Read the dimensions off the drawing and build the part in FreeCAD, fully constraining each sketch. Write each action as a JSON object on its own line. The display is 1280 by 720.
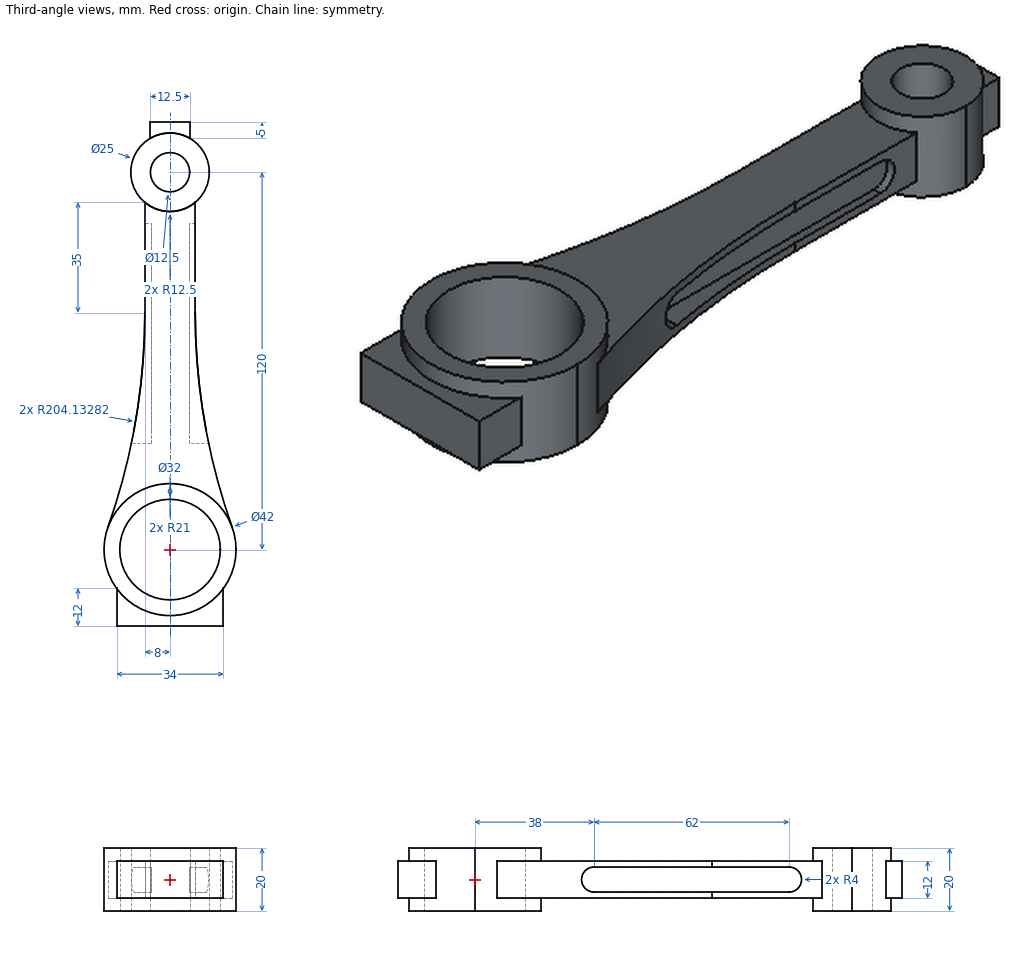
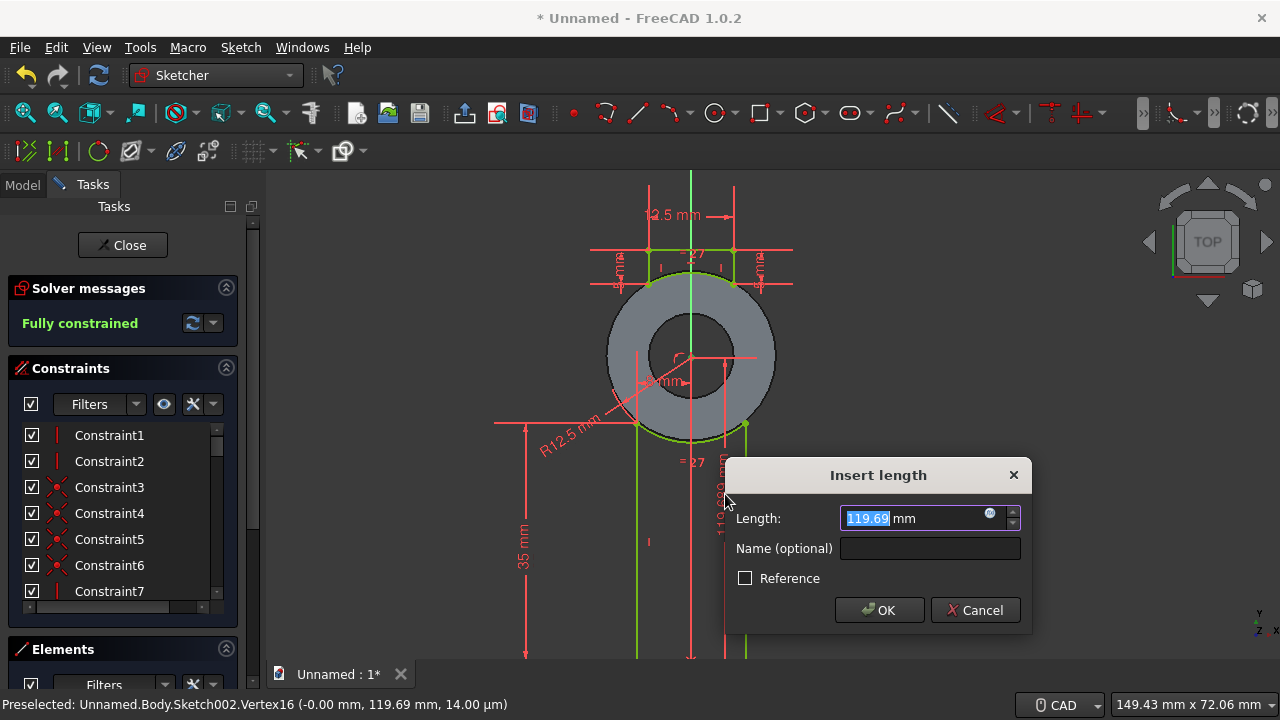
{"action": "type", "text": "120"}
{"action": "key", "text": "Return"}
{"action": "key", "text": "Escape"}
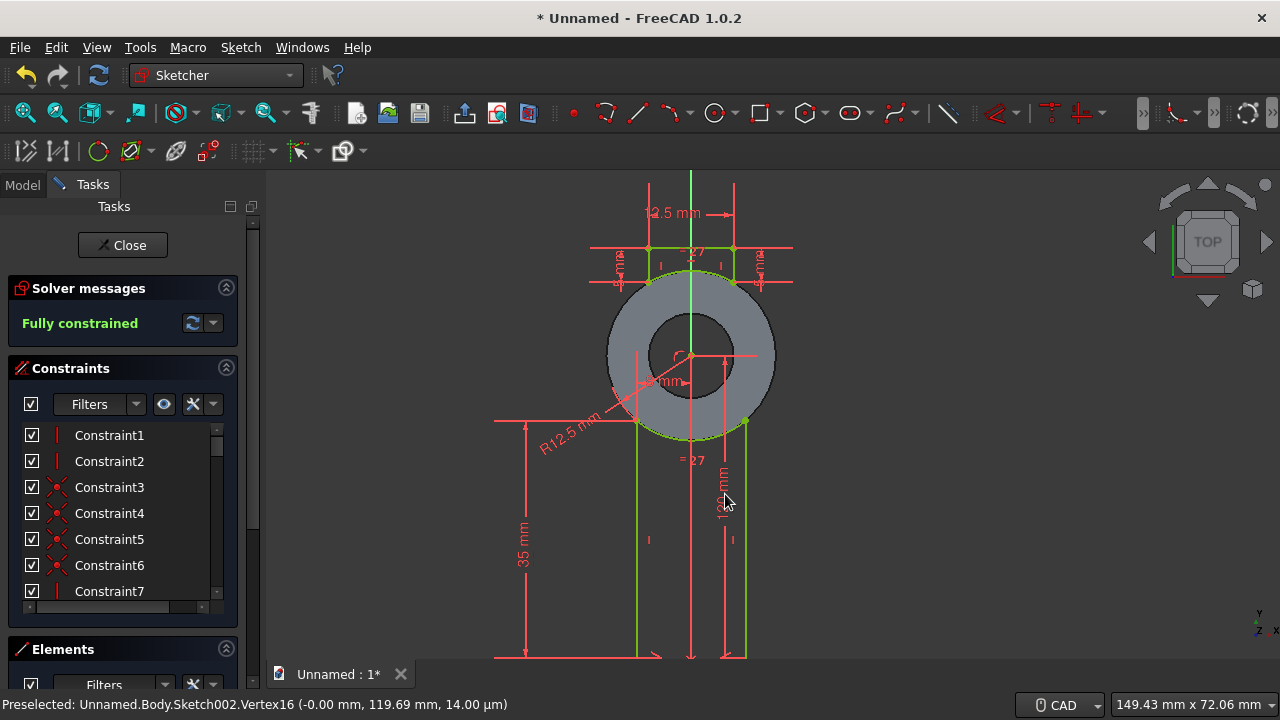
{"action": "left_click", "coordinate": [123, 245]}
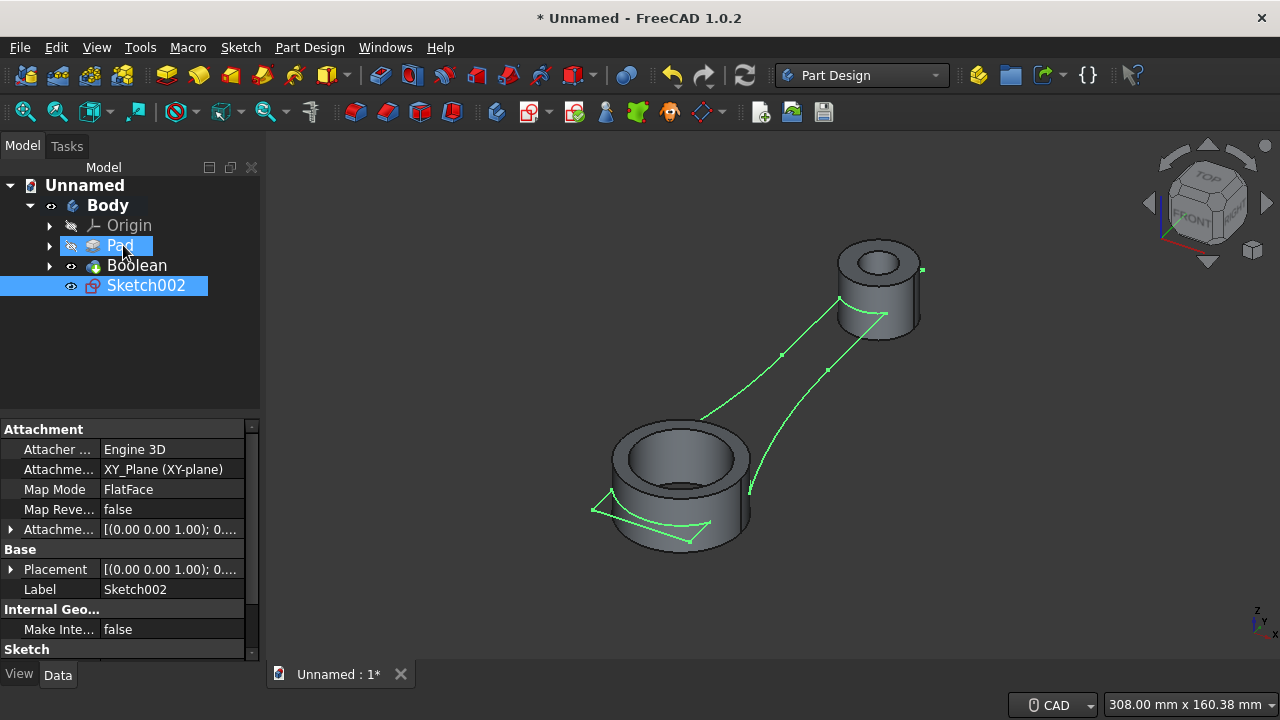
{"action": "left_click", "coordinate": [168, 76]}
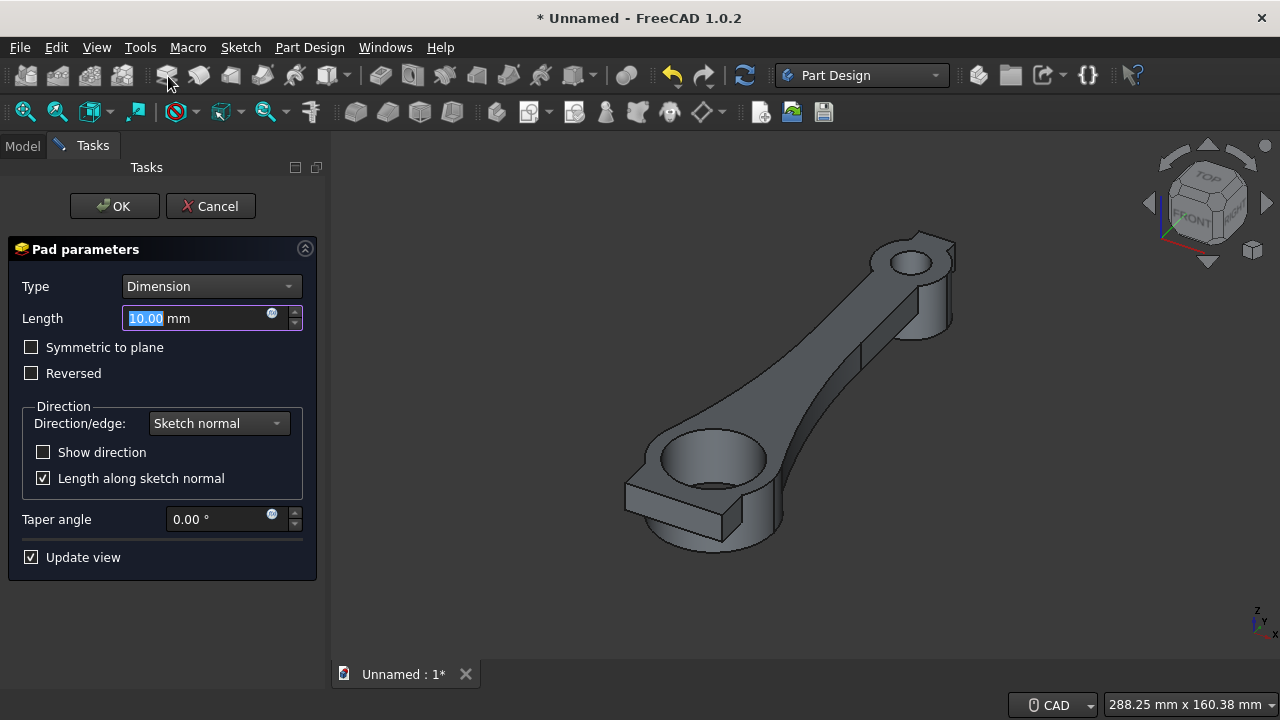
{"action": "type", "text": "12"}
{"action": "key", "text": "Tab"}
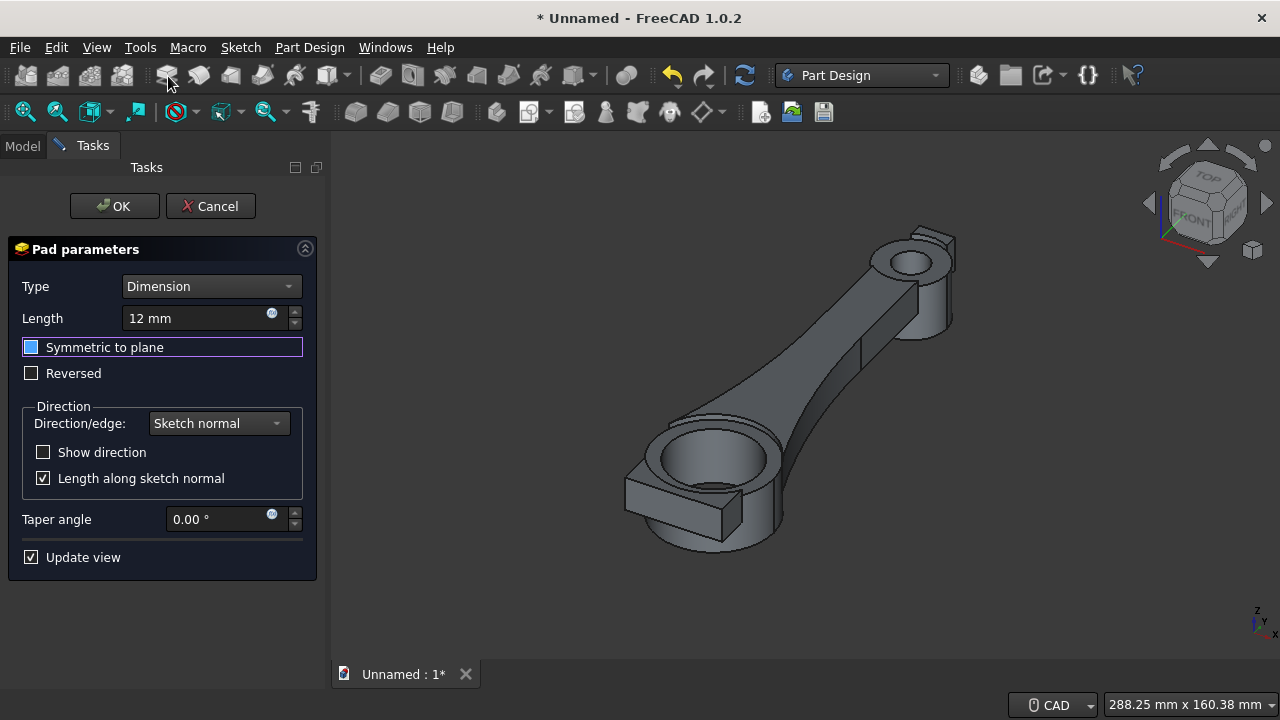
{"action": "left_click", "coordinate": [30, 347]}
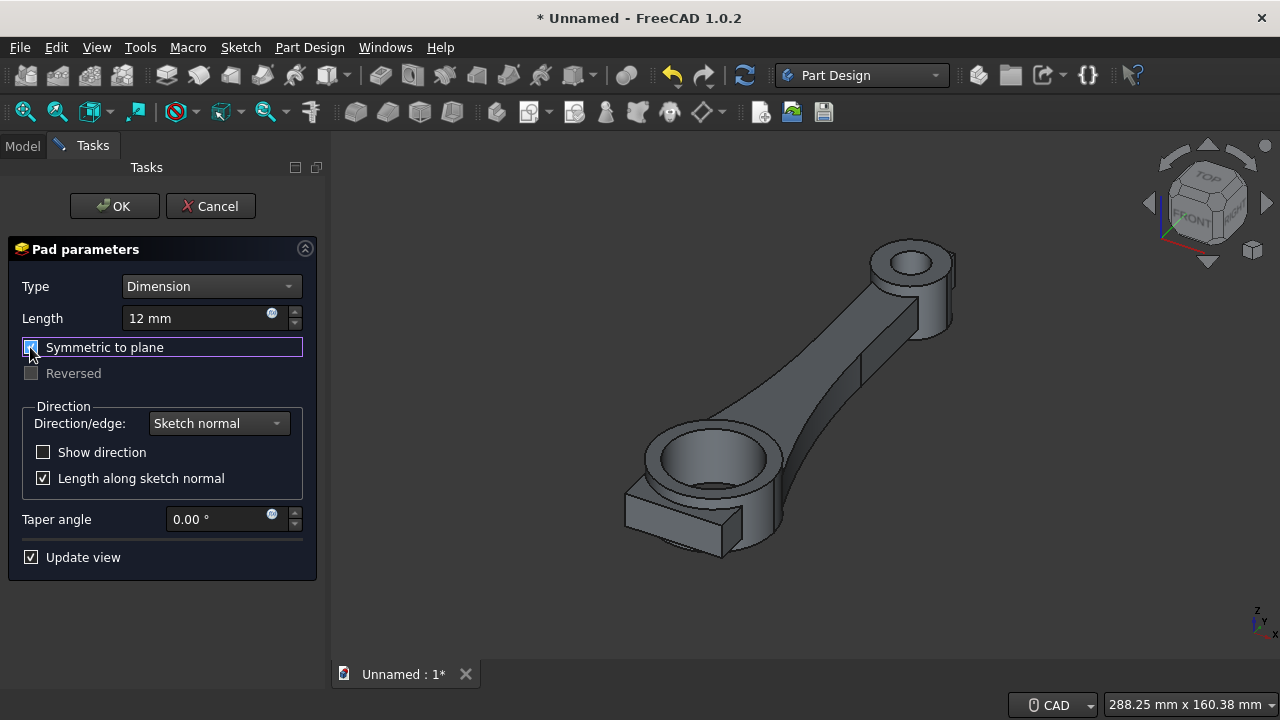
{"action": "left_click", "coordinate": [115, 206]}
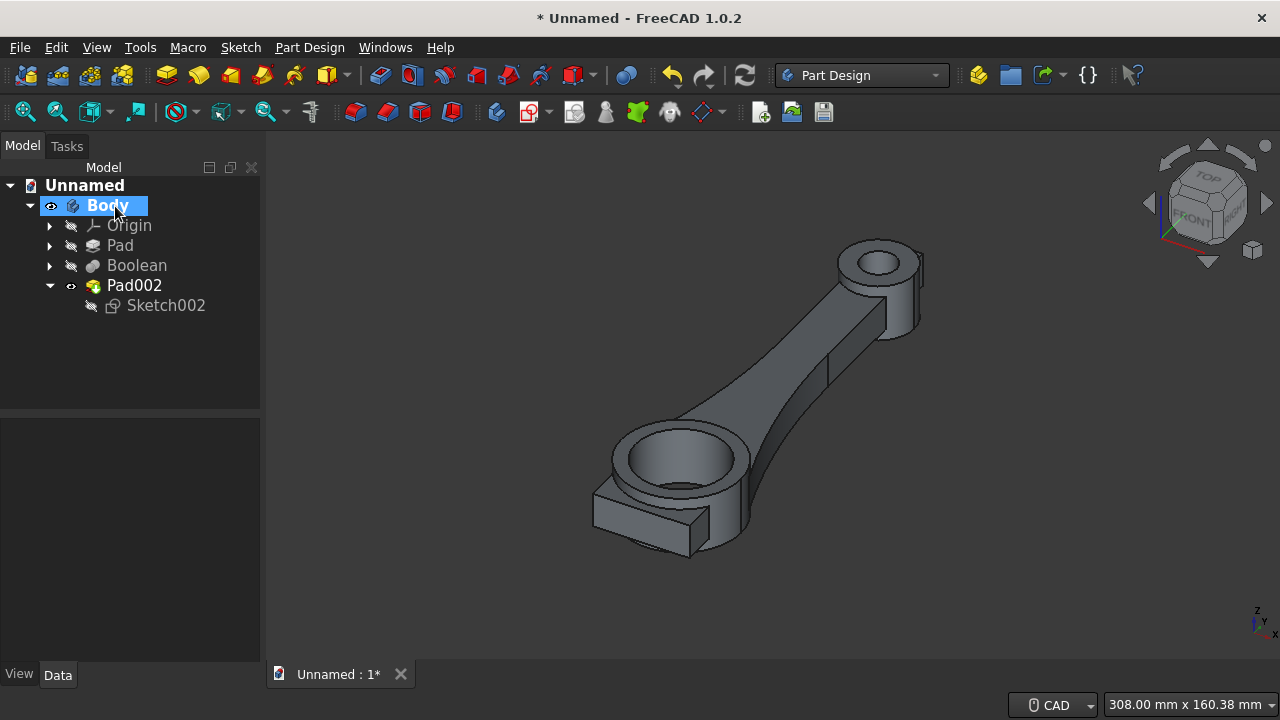
{"action": "left_click", "coordinate": [50, 226]}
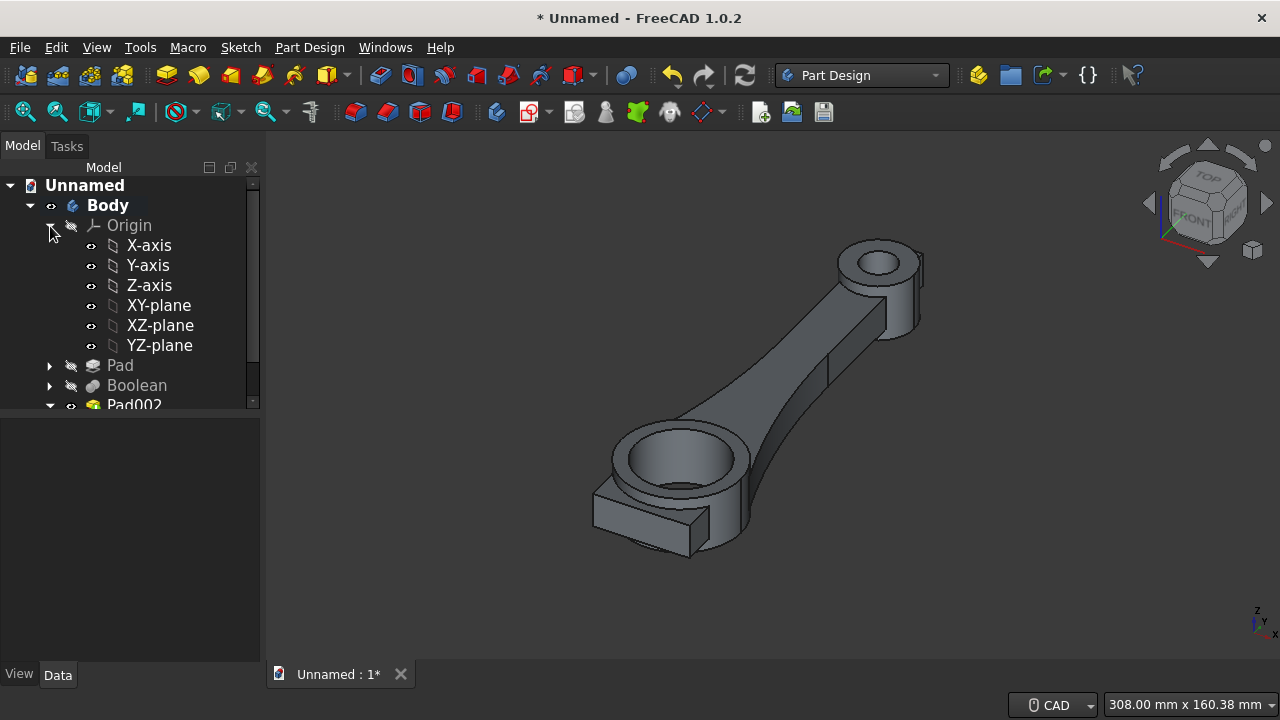
{"action": "left_click", "coordinate": [136, 346]}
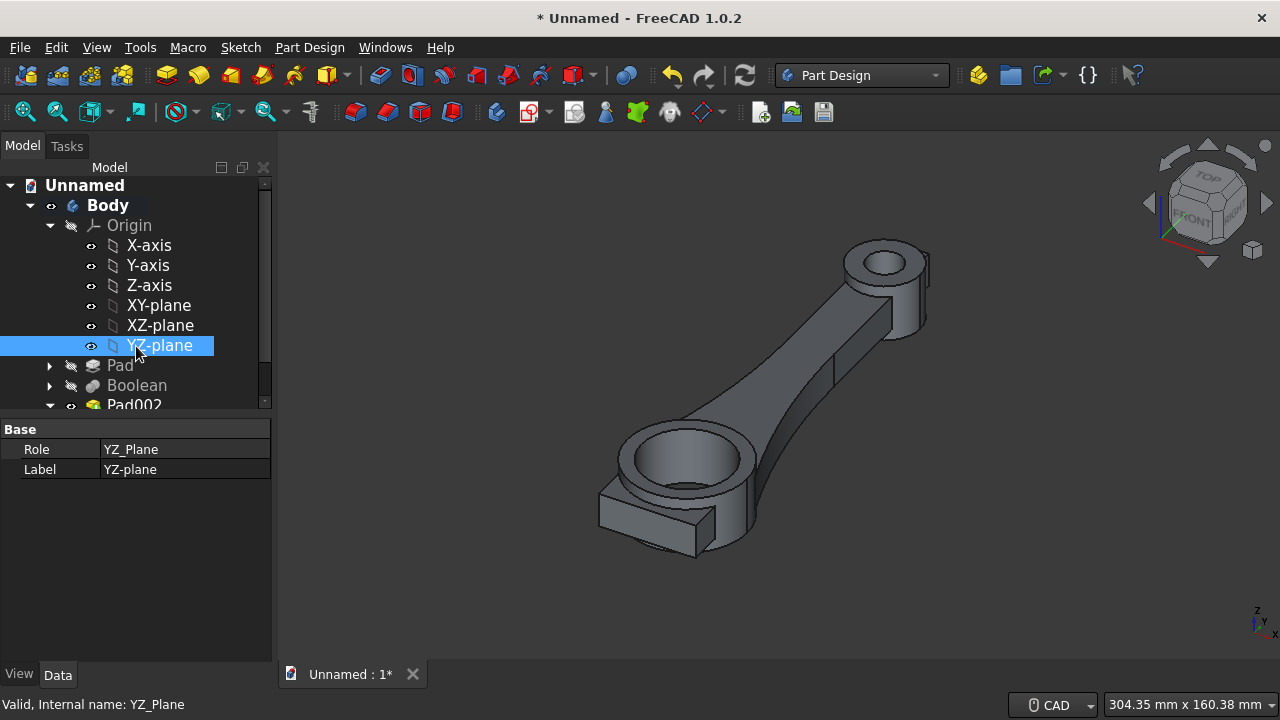
{"action": "left_click", "coordinate": [702, 112]}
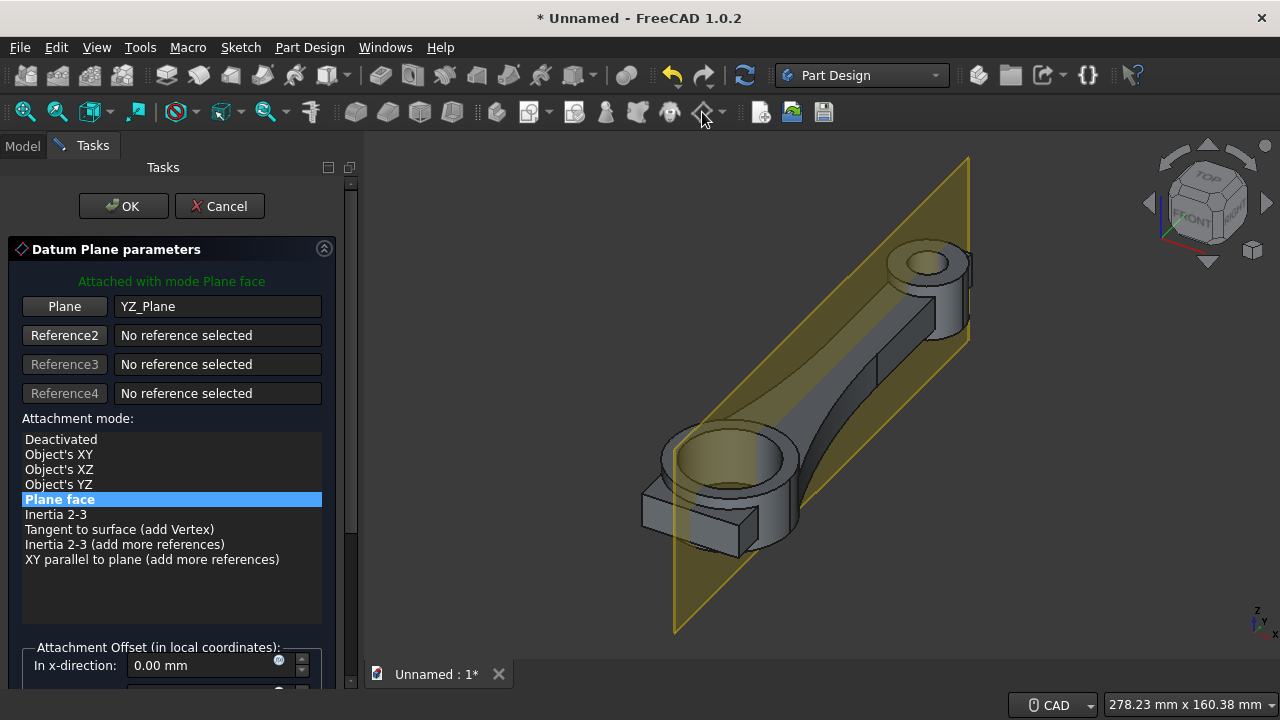
{"action": "scroll", "coordinate": [351, 432], "scroll_direction": "down", "scroll_amount": 2}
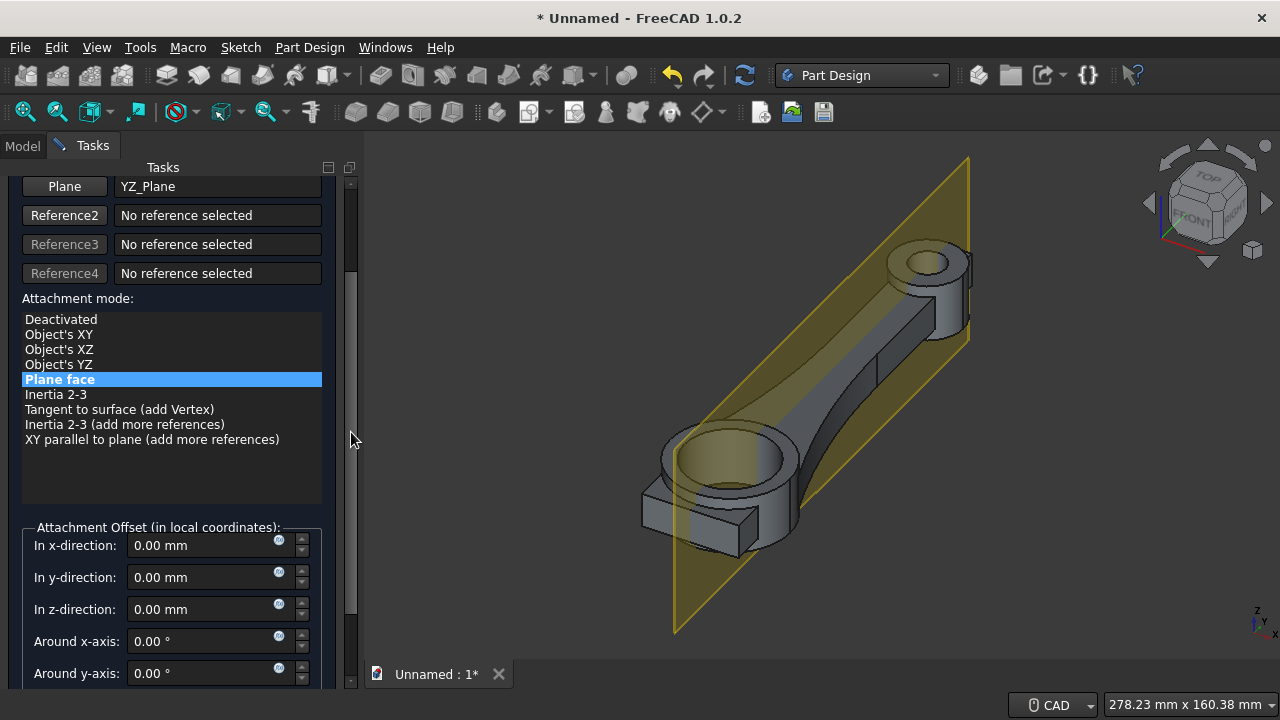
{"action": "triple_click", "coordinate": [210, 609]}